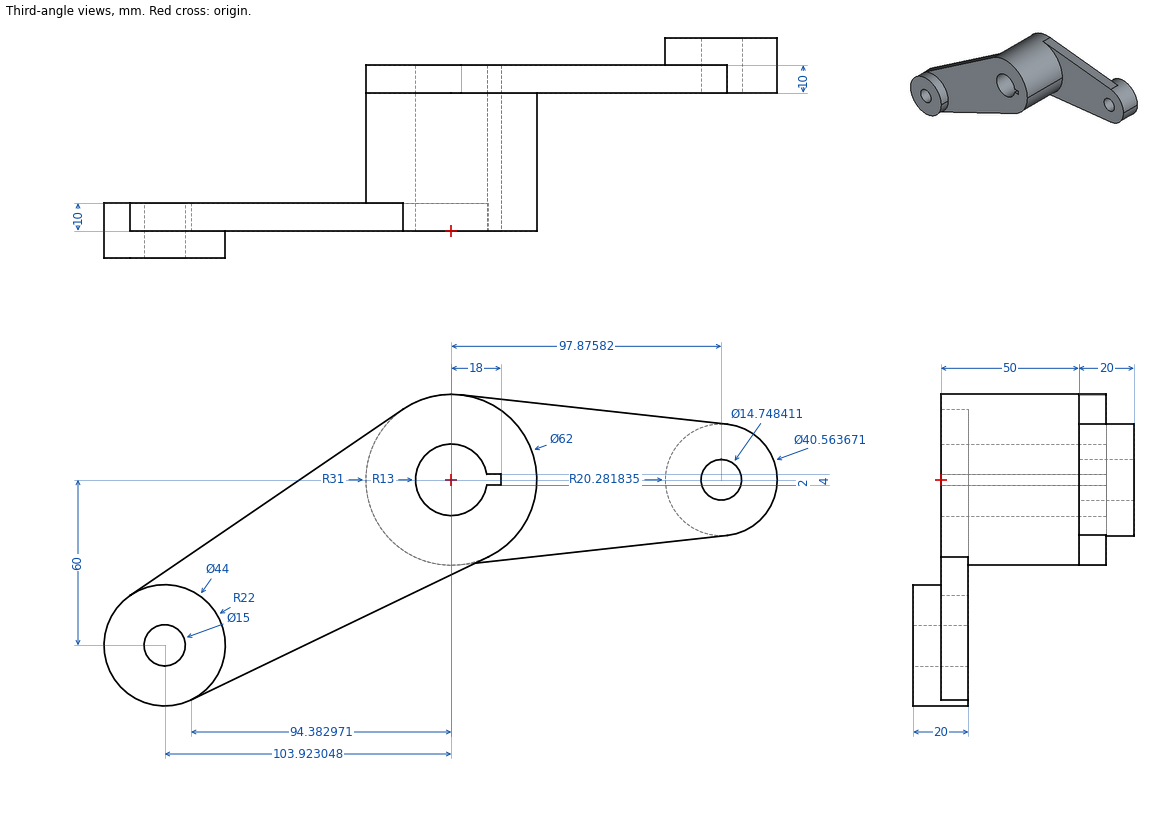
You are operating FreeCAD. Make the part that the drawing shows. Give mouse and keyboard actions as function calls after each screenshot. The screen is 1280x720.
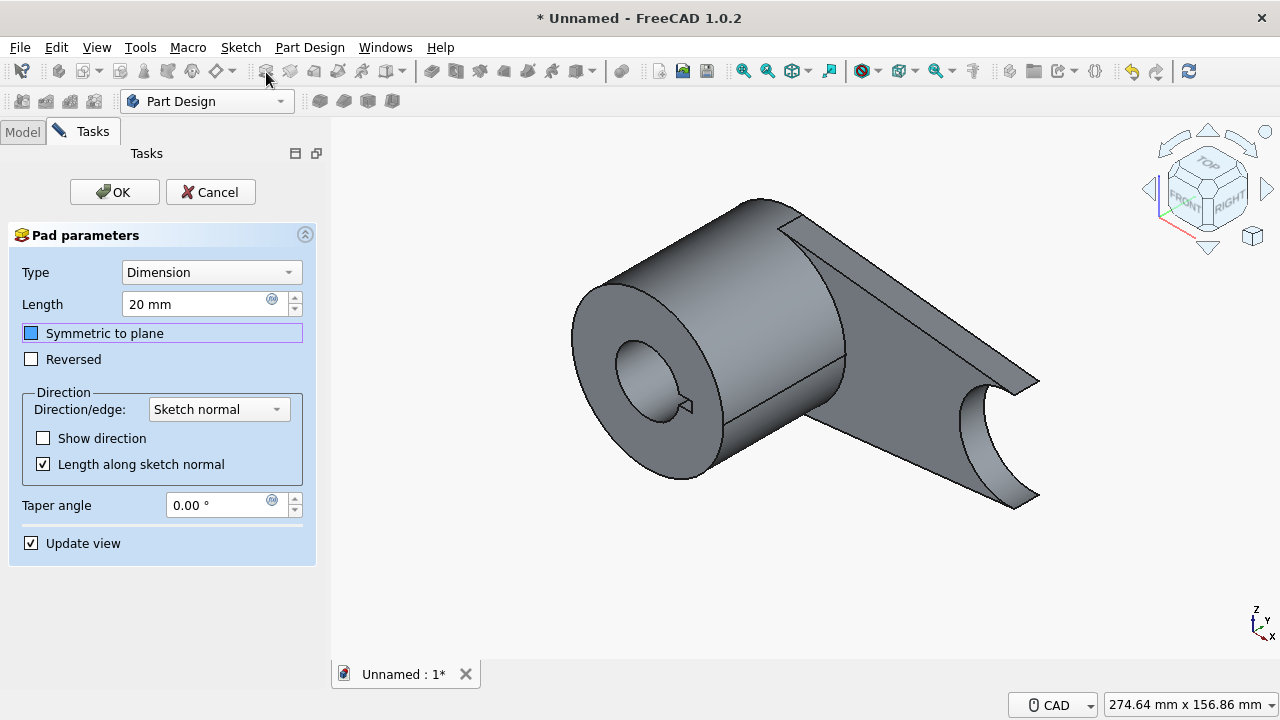
click(30, 359)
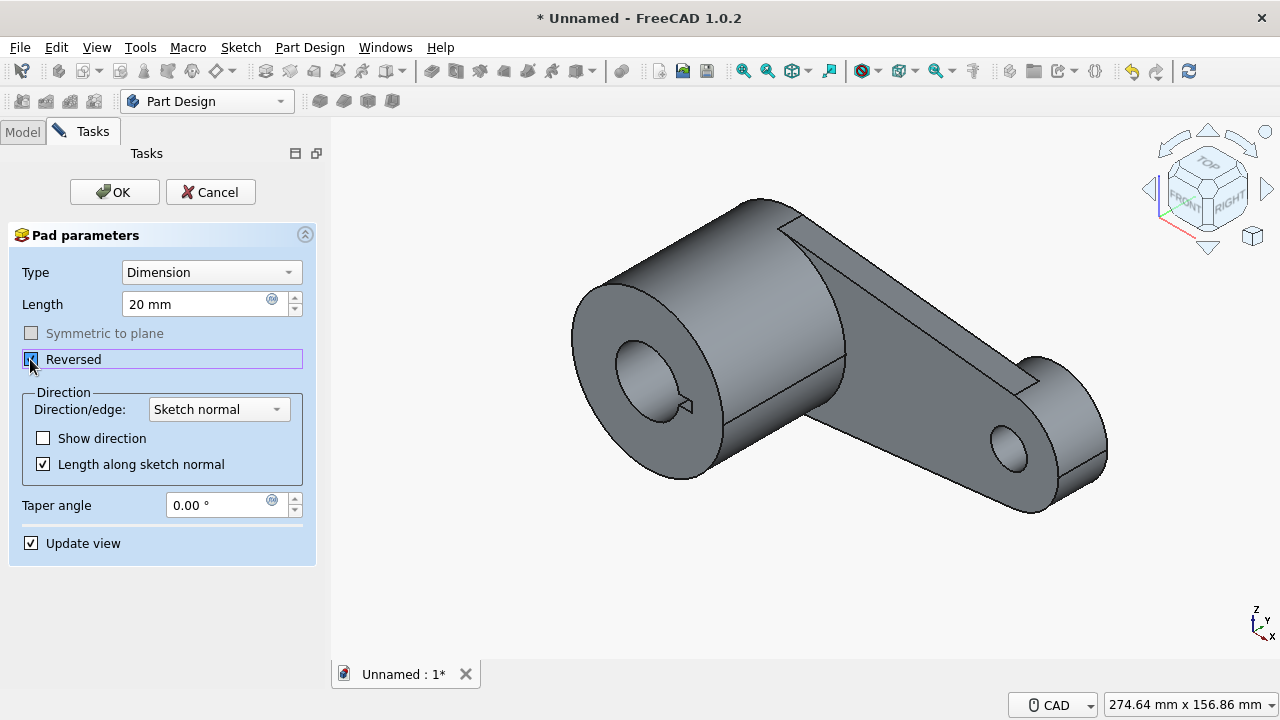
click(115, 192)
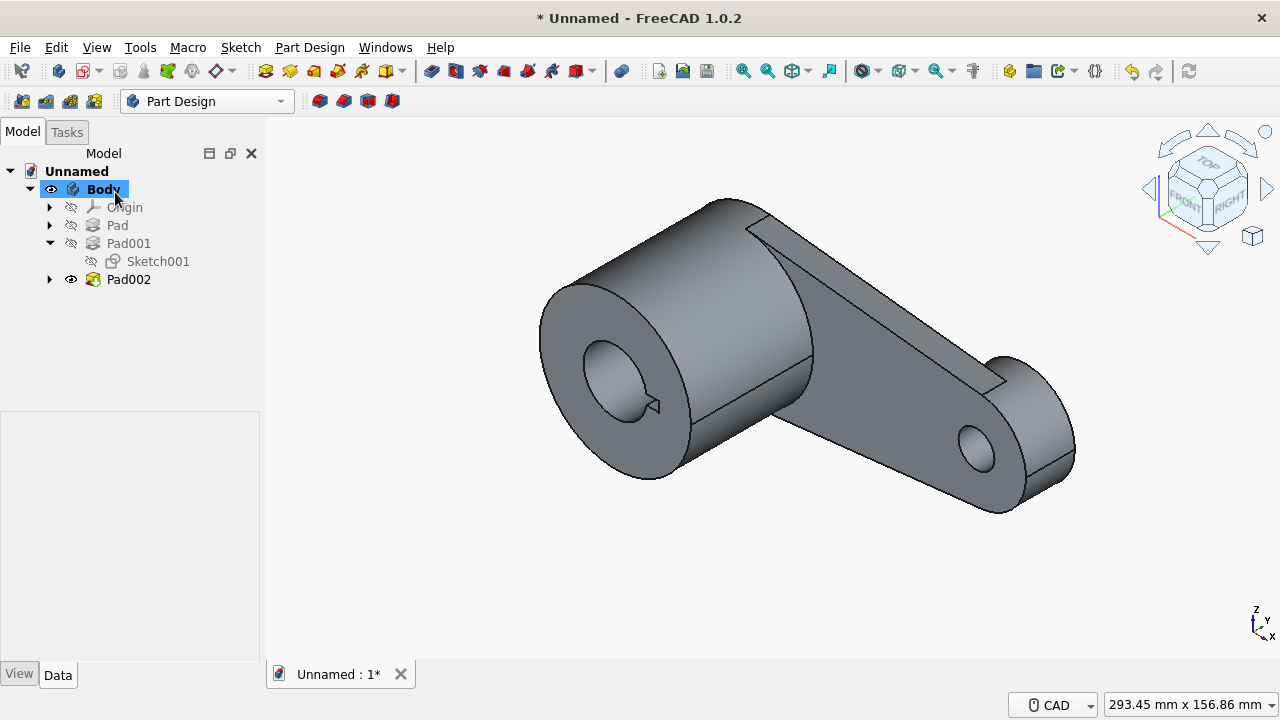
click(84, 72)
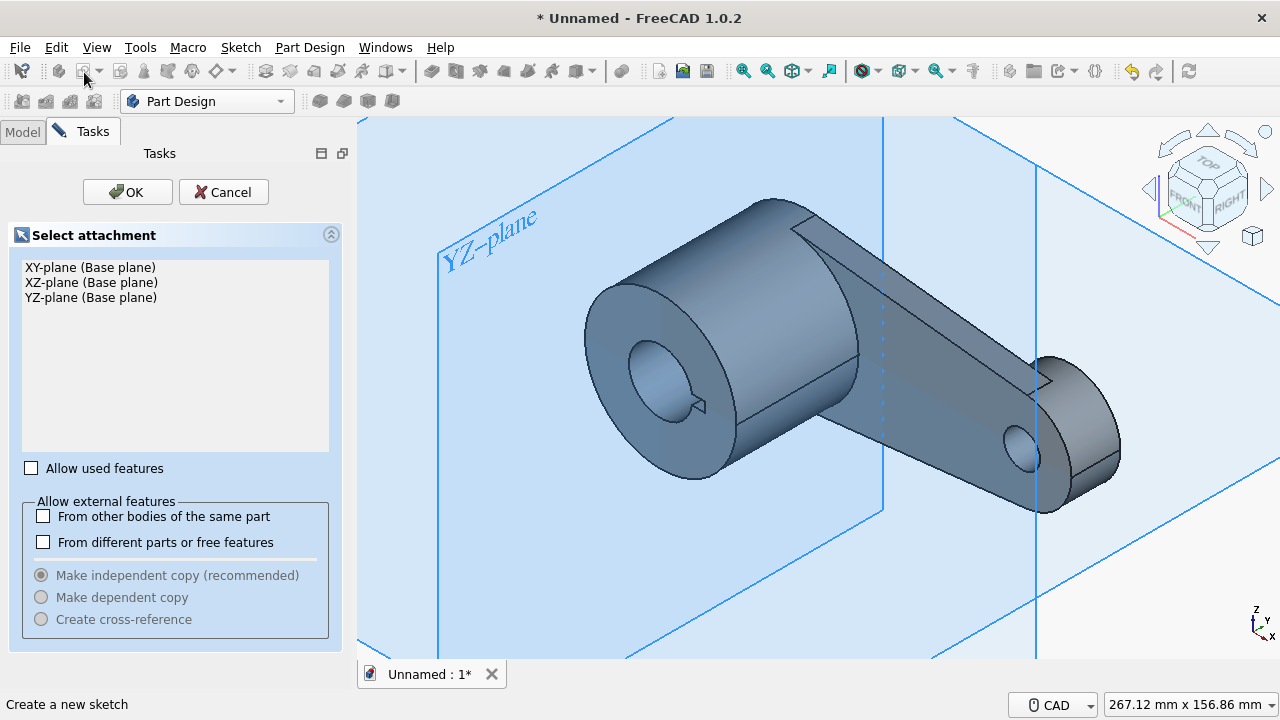
click(82, 282)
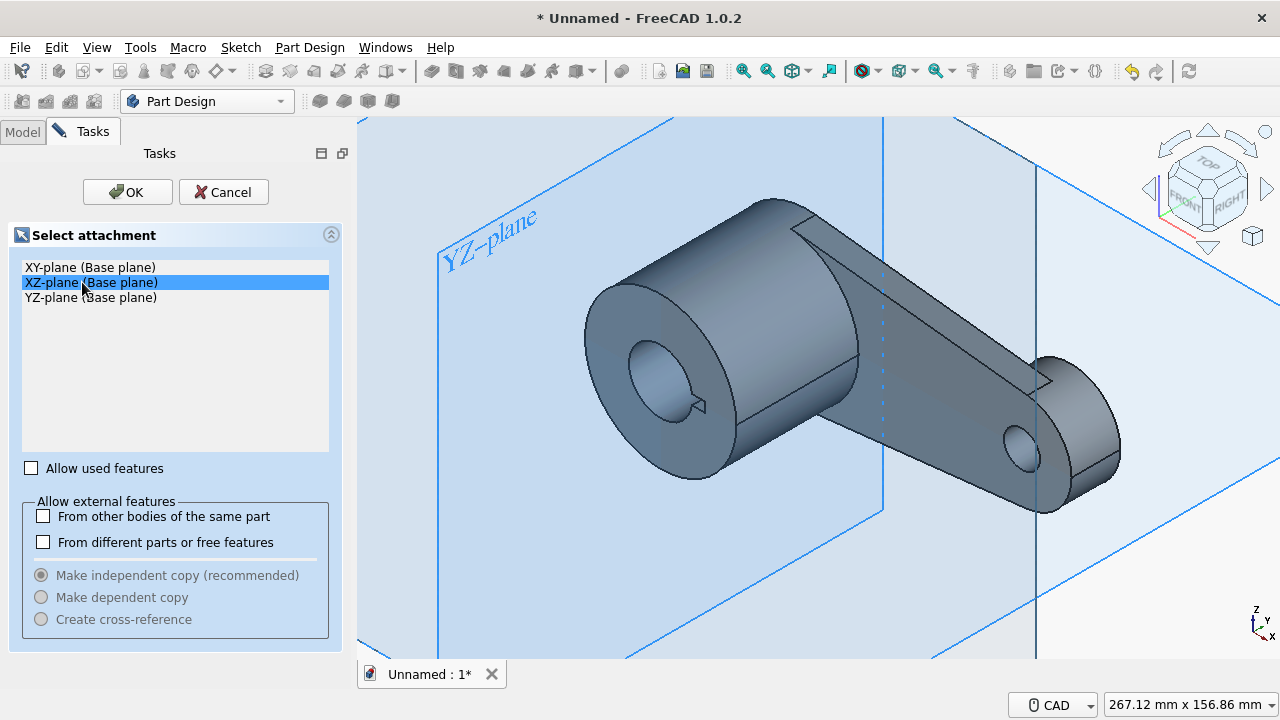
click(128, 192)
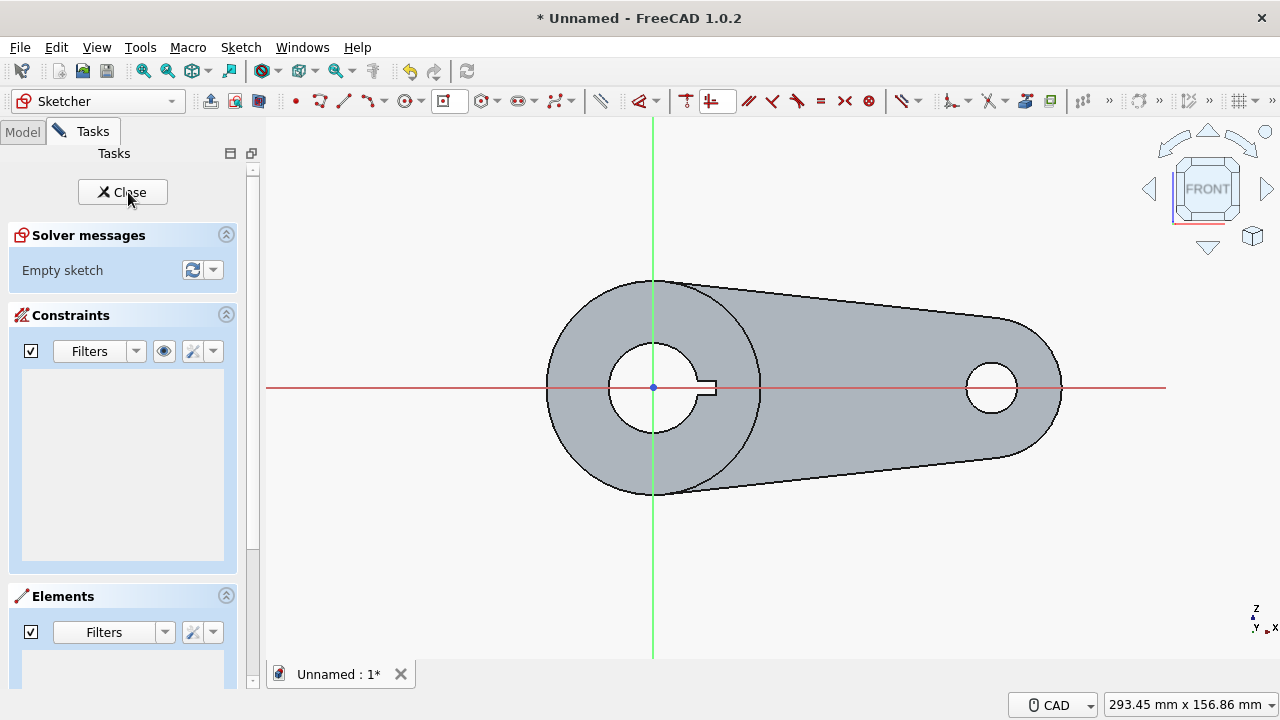
scroll(1115, 145, down, 1)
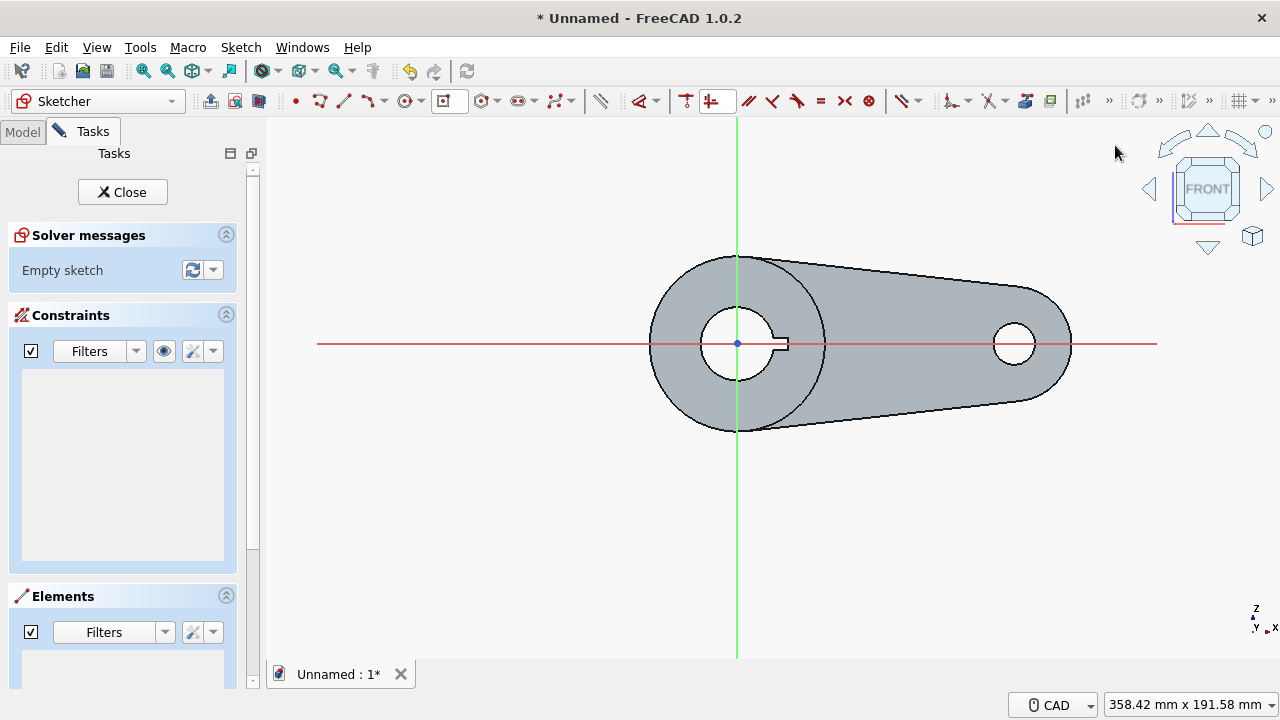
key(g)
key(l)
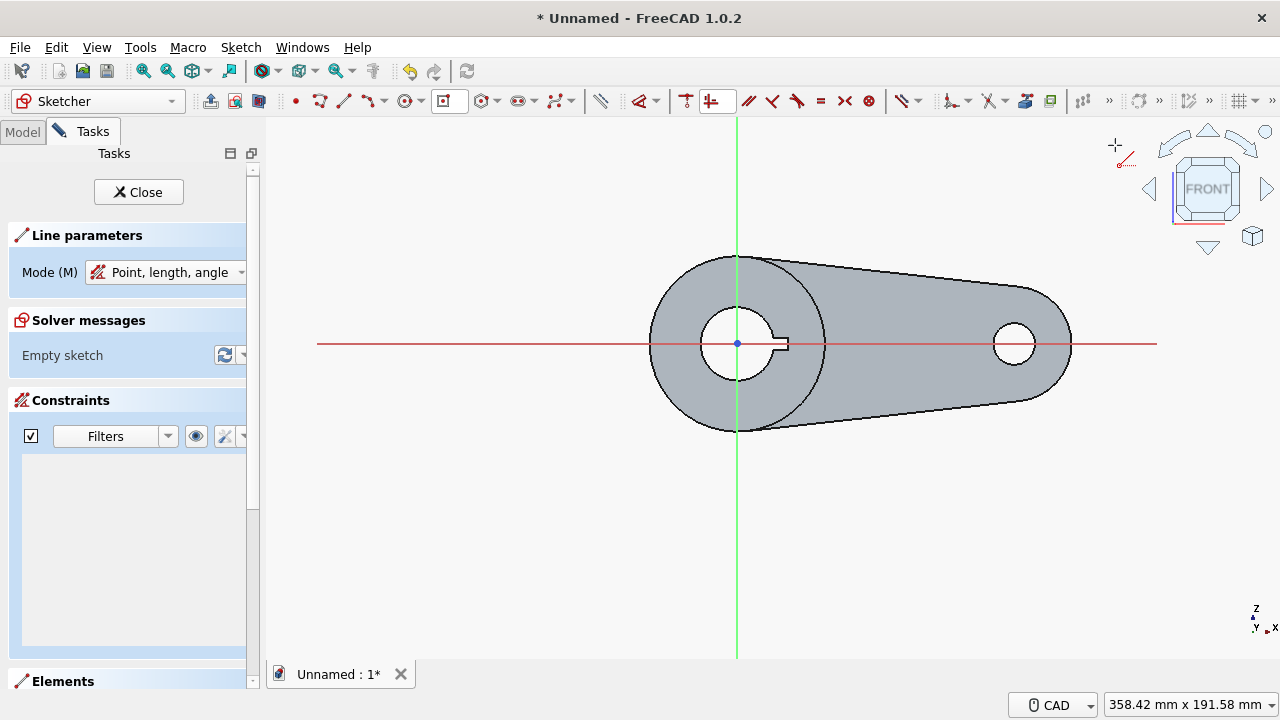
click(688, 272)
click(408, 462)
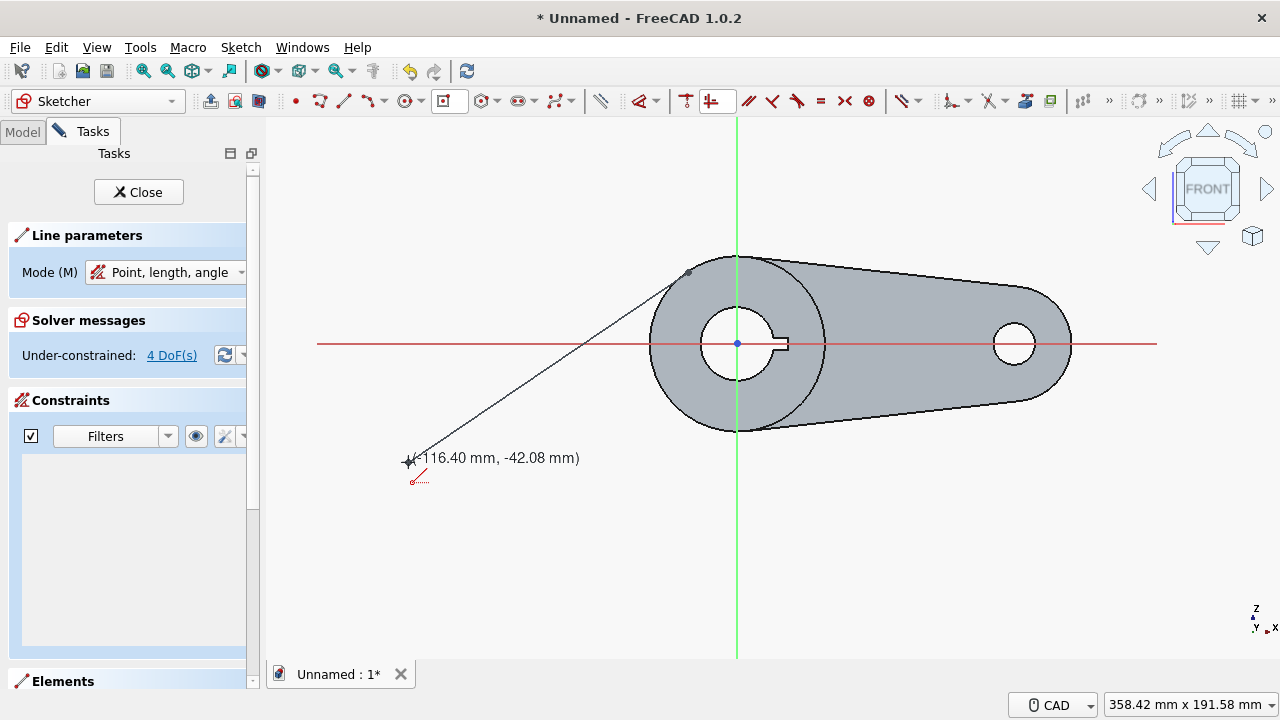
click(470, 570)
click(775, 423)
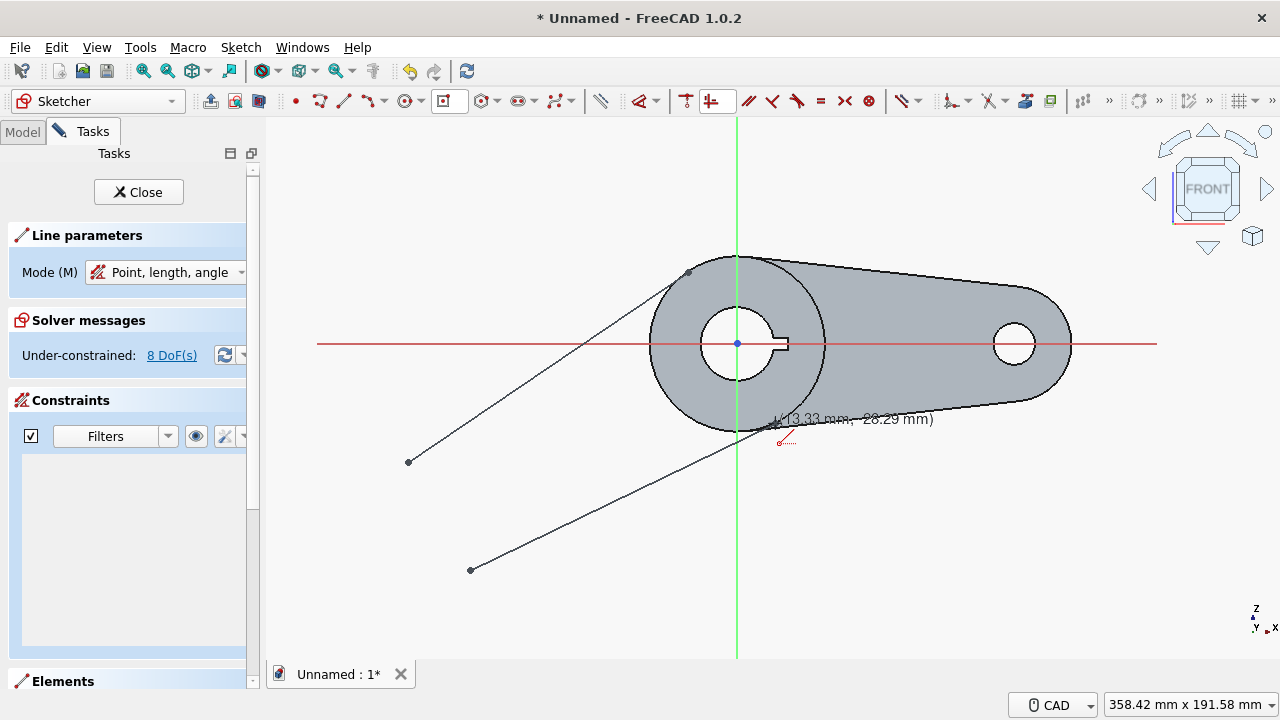
click(368, 102)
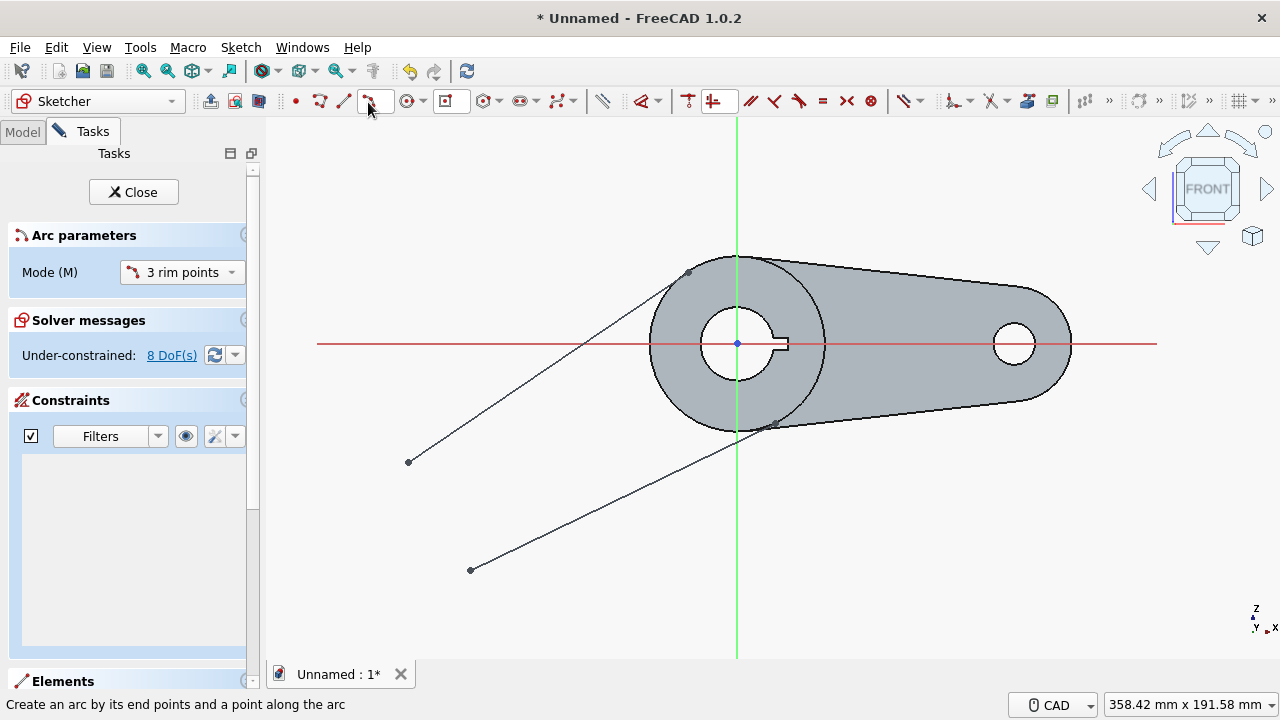
click(408, 463)
click(470, 571)
click(497, 483)